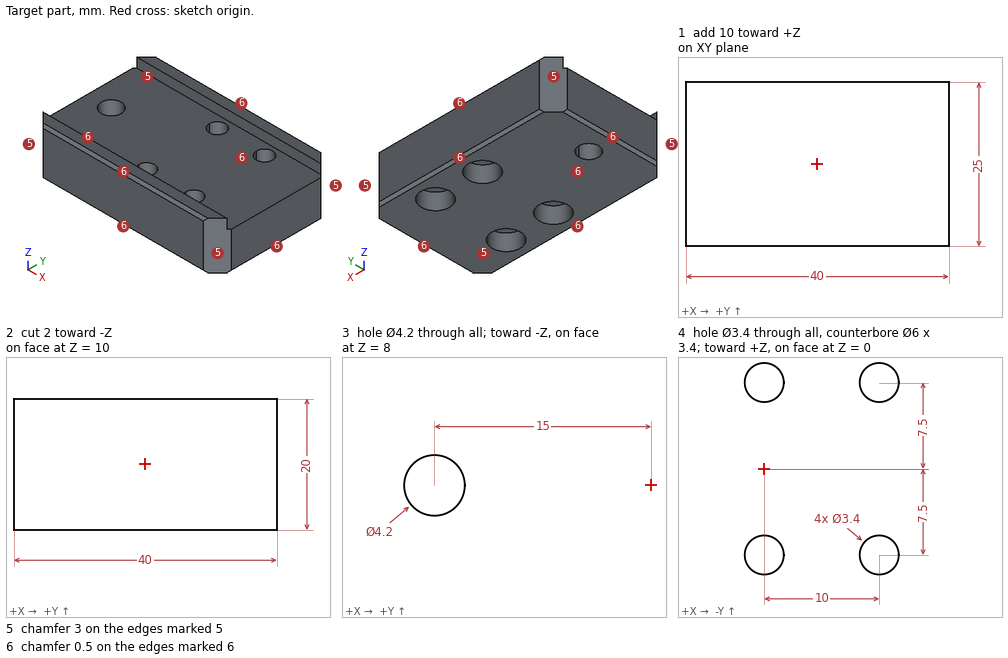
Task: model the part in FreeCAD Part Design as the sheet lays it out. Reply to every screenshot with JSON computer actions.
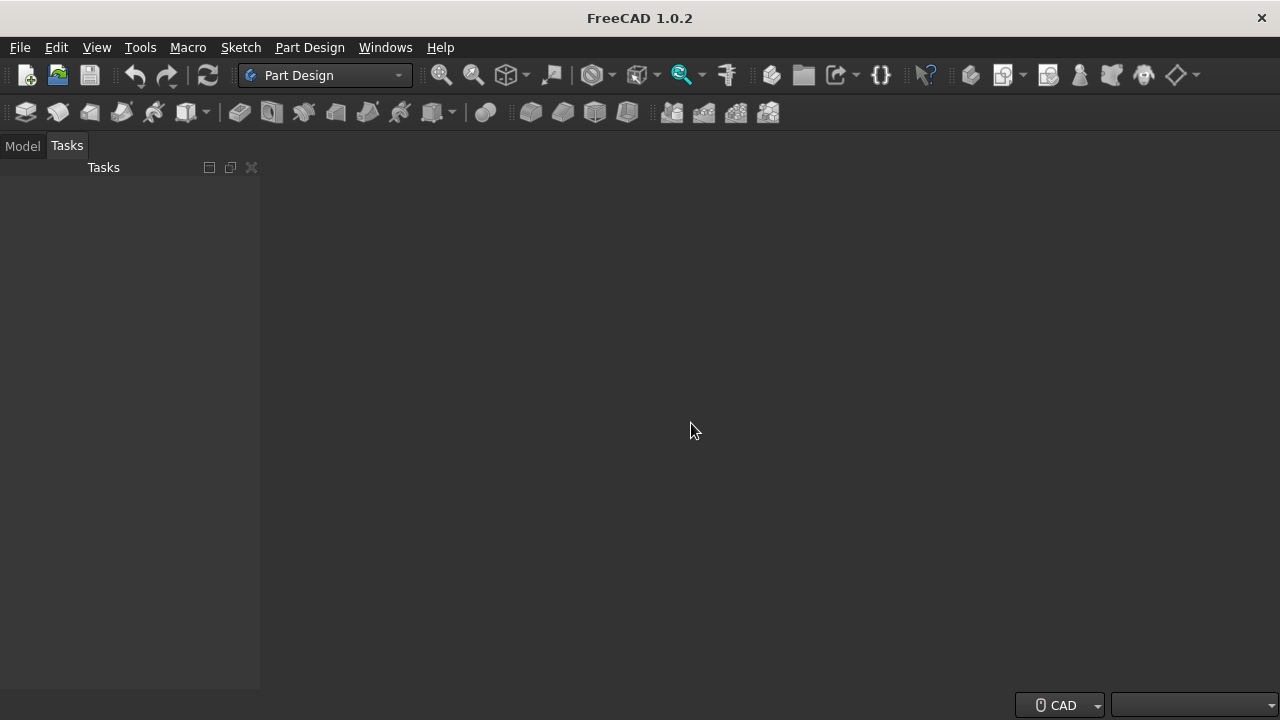
{"action": "left_click", "coordinate": [26, 76]}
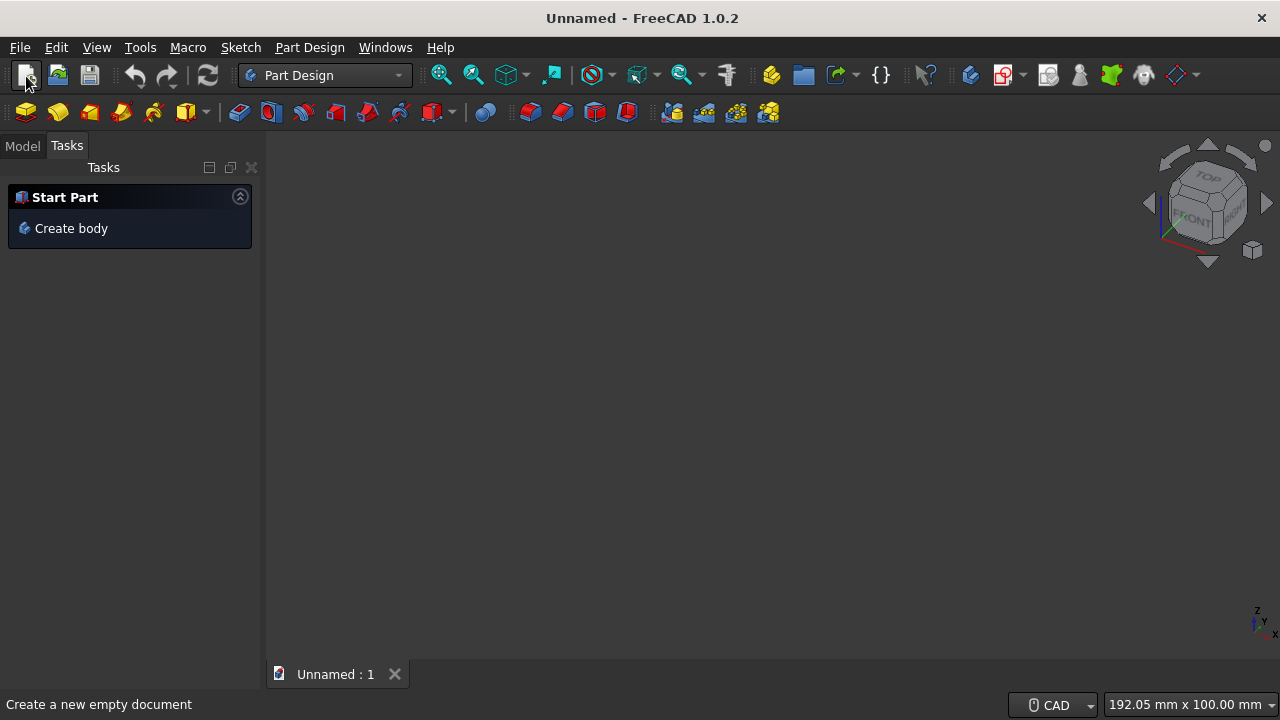
{"action": "left_click", "coordinate": [1004, 76]}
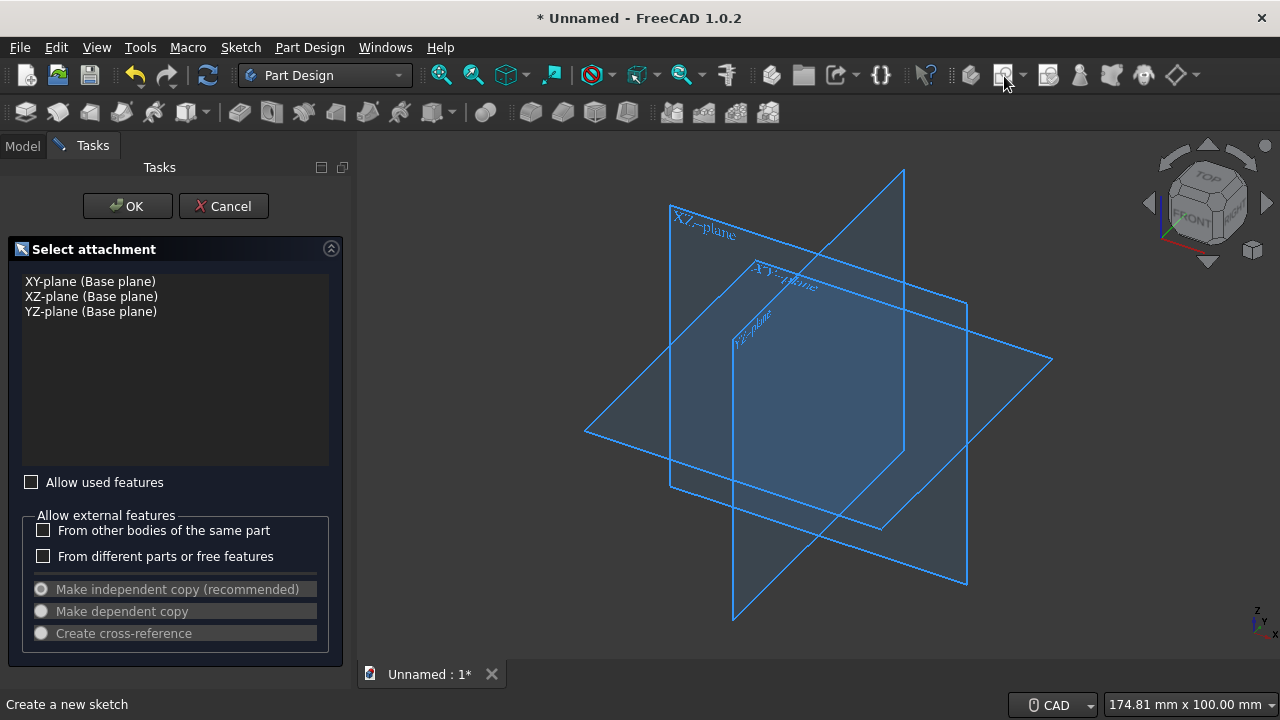
{"action": "left_click", "coordinate": [82, 282]}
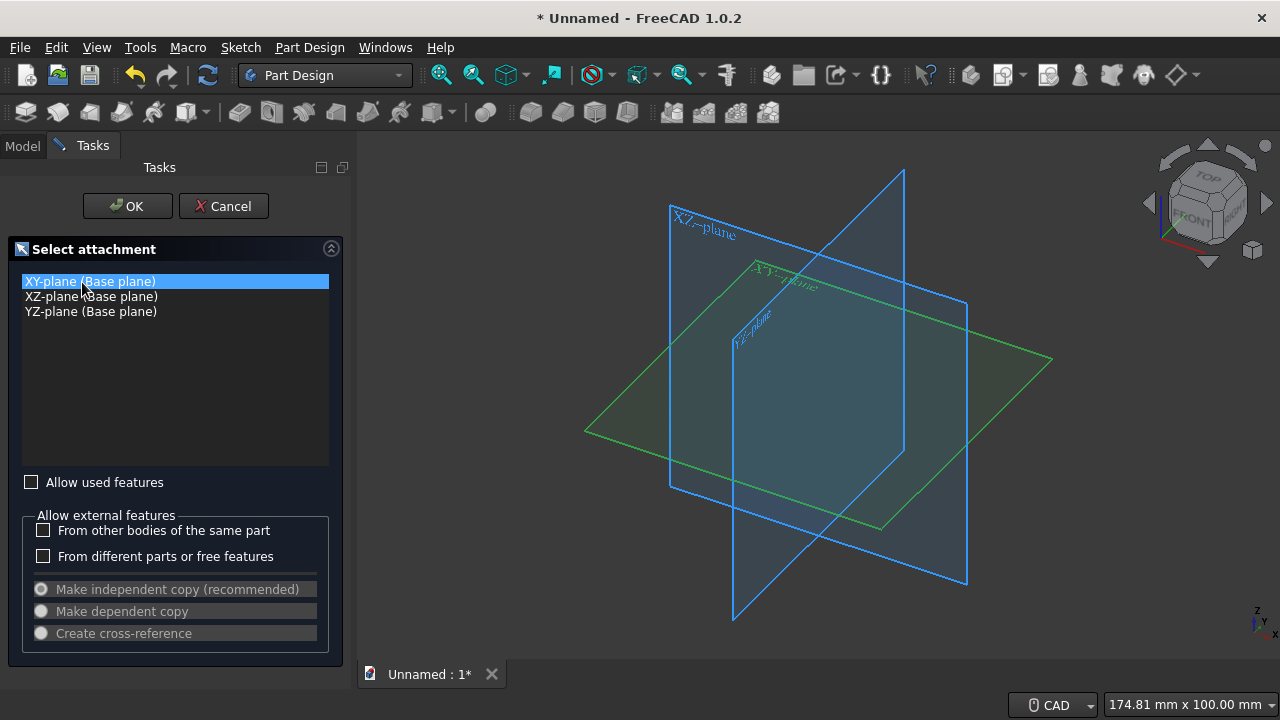
{"action": "left_click", "coordinate": [128, 206]}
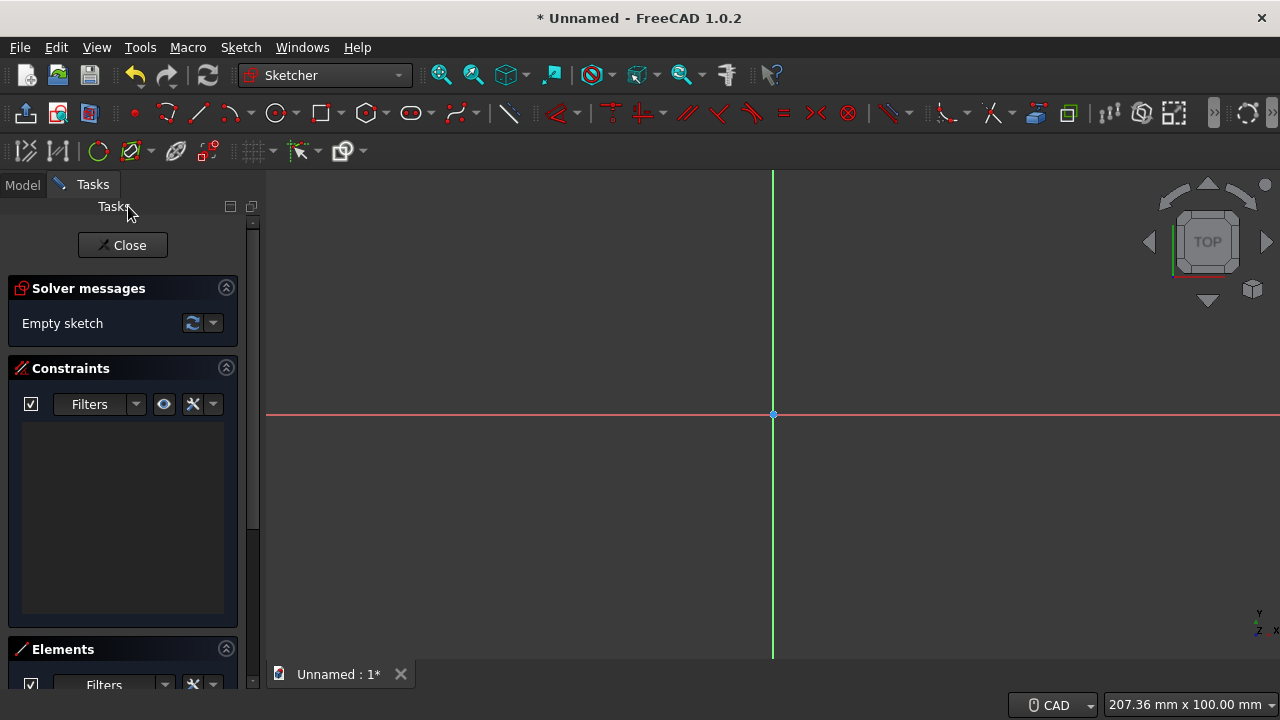
{"action": "scroll", "coordinate": [813, 415], "scroll_direction": "up", "scroll_amount": 5}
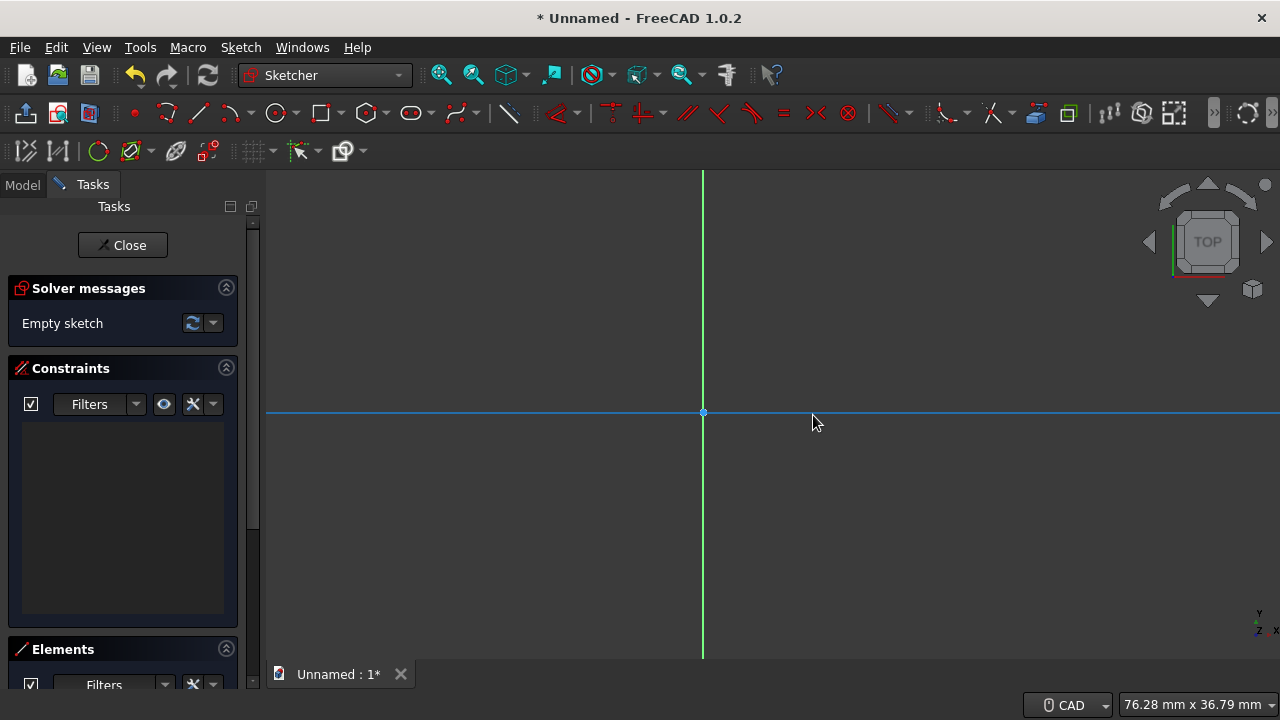
{"action": "left_click", "coordinate": [344, 114]}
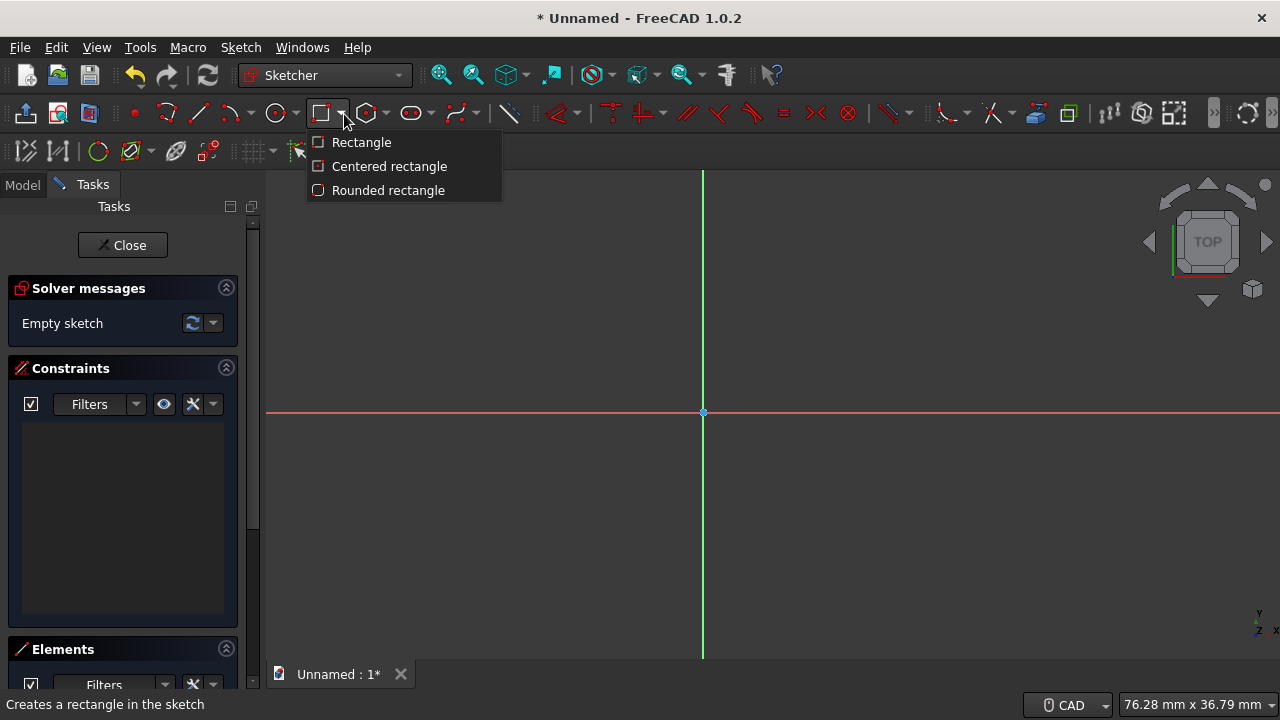
{"action": "left_click", "coordinate": [404, 166]}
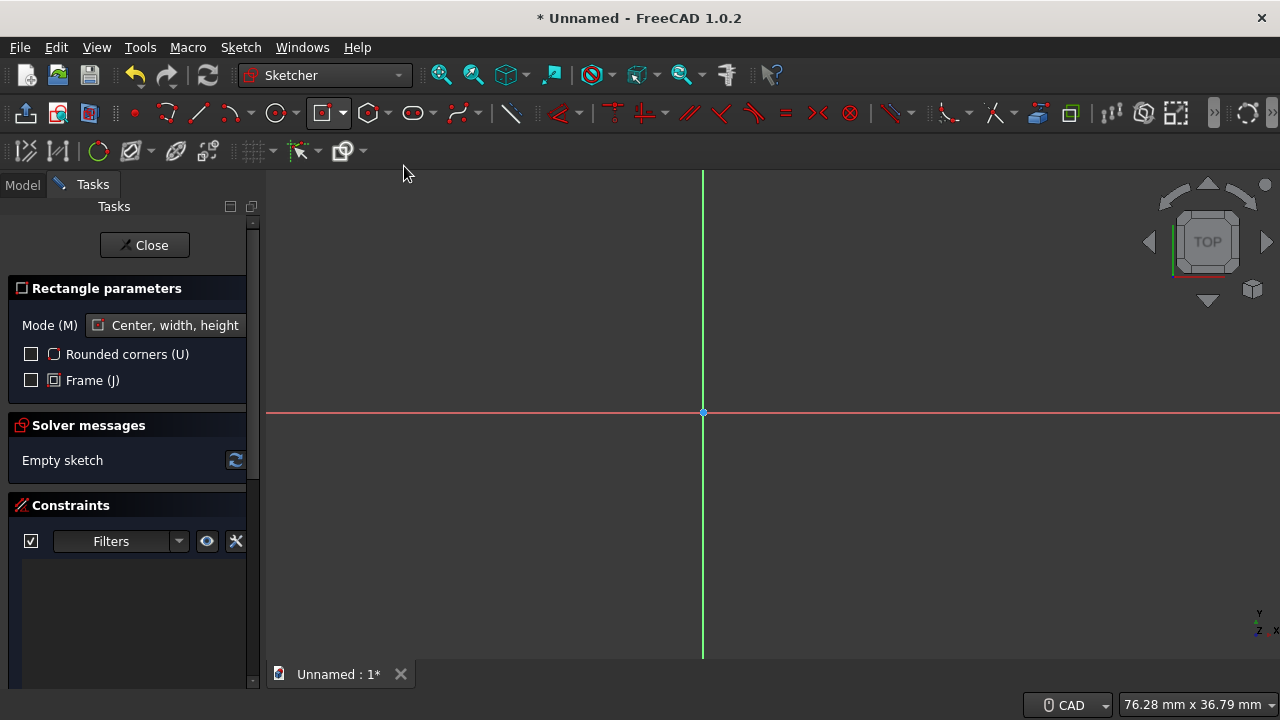
{"action": "left_click", "coordinate": [703, 413]}
{"action": "left_click", "coordinate": [969, 247]}
{"action": "key", "text": "Escape"}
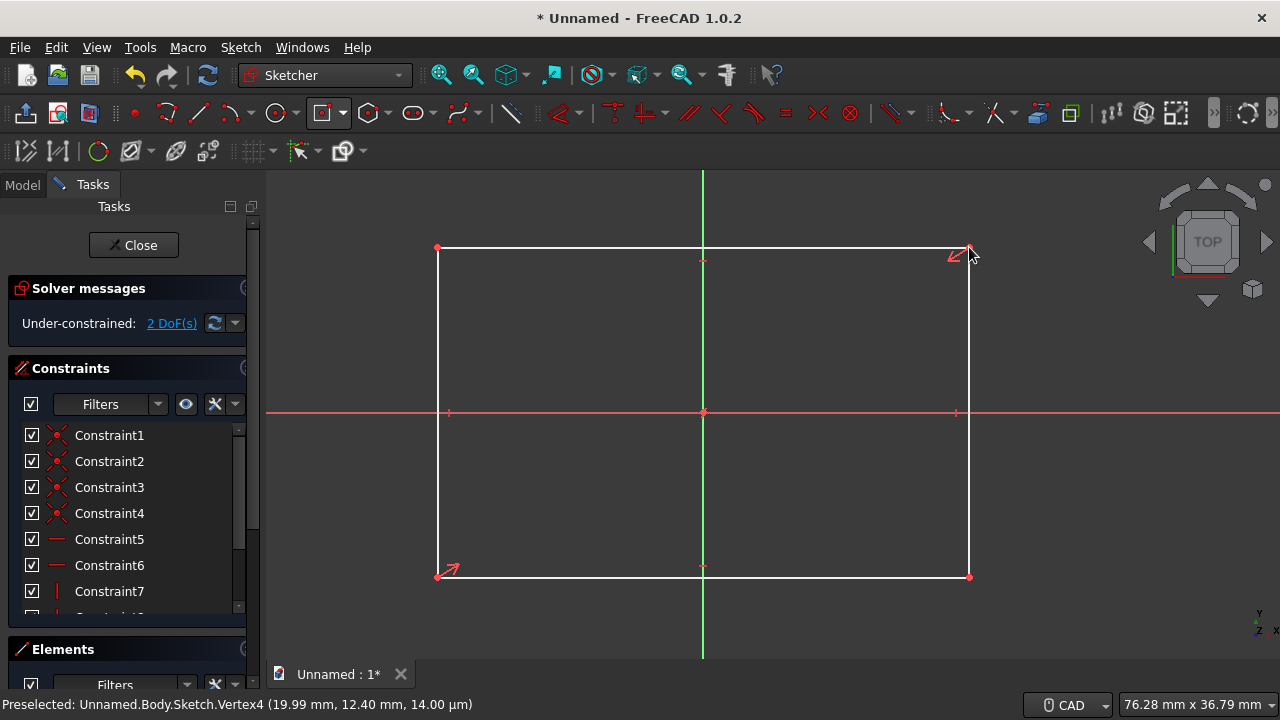
{"action": "left_click", "coordinate": [558, 114]}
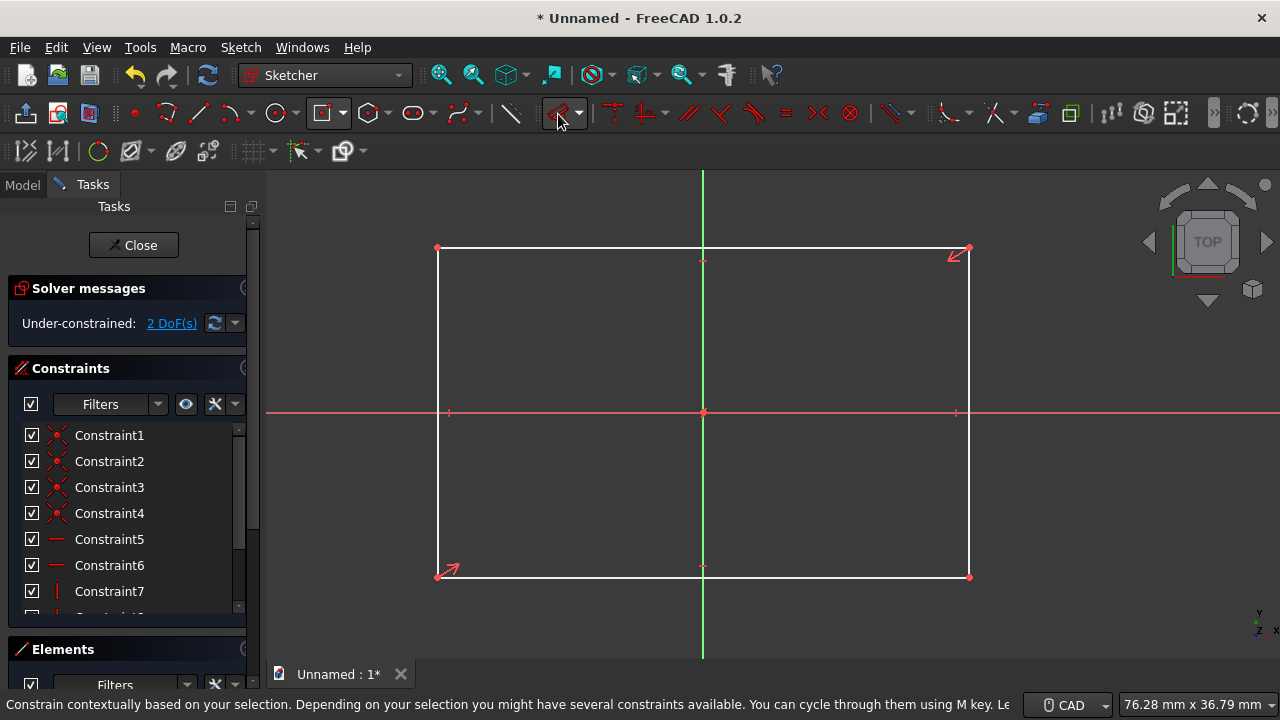
{"action": "left_click", "coordinate": [597, 578]}
{"action": "left_click", "coordinate": [581, 612]}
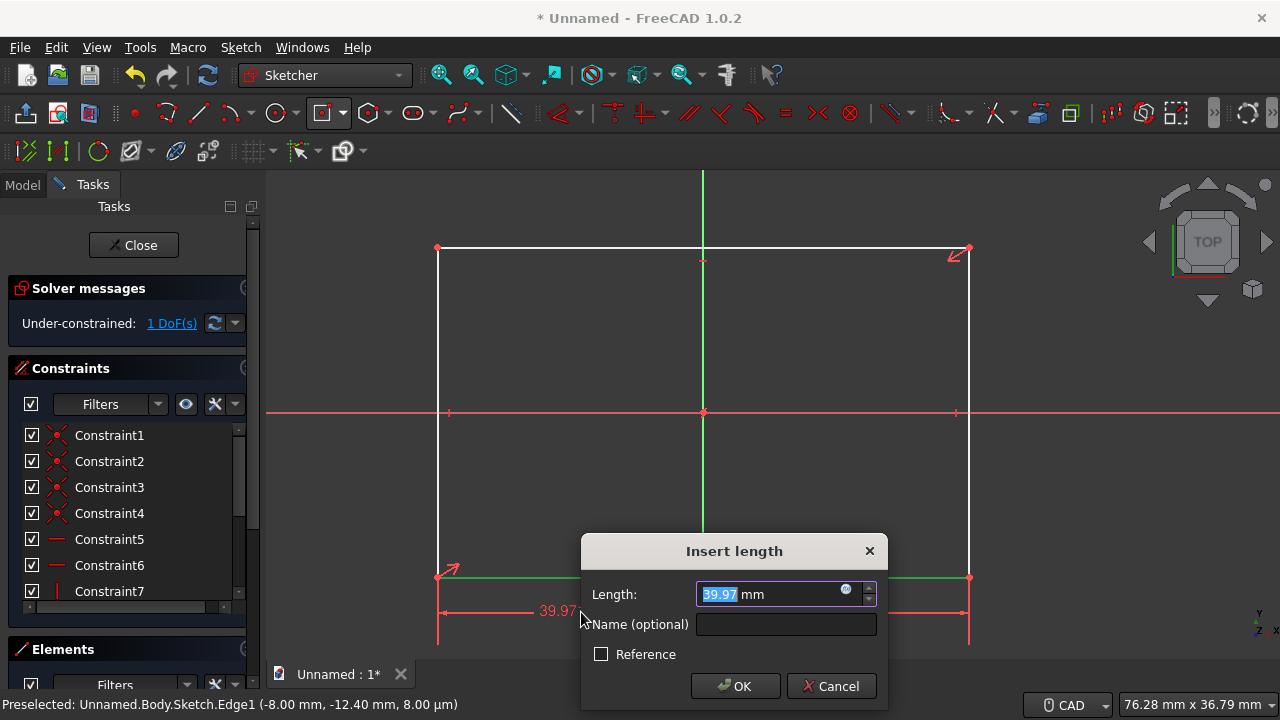
{"action": "type", "text": "40"}
{"action": "key", "text": "Return"}